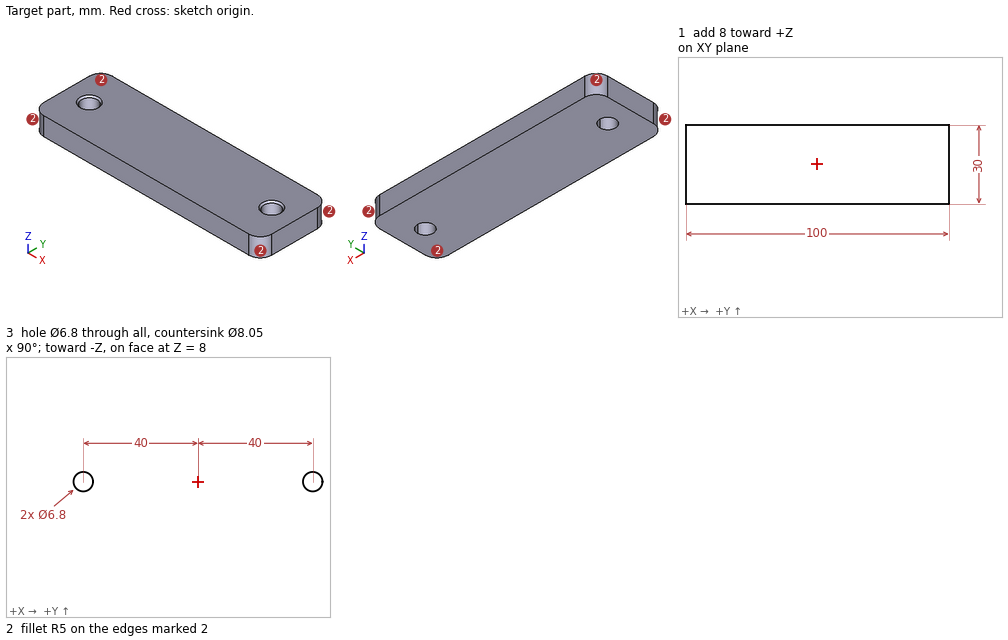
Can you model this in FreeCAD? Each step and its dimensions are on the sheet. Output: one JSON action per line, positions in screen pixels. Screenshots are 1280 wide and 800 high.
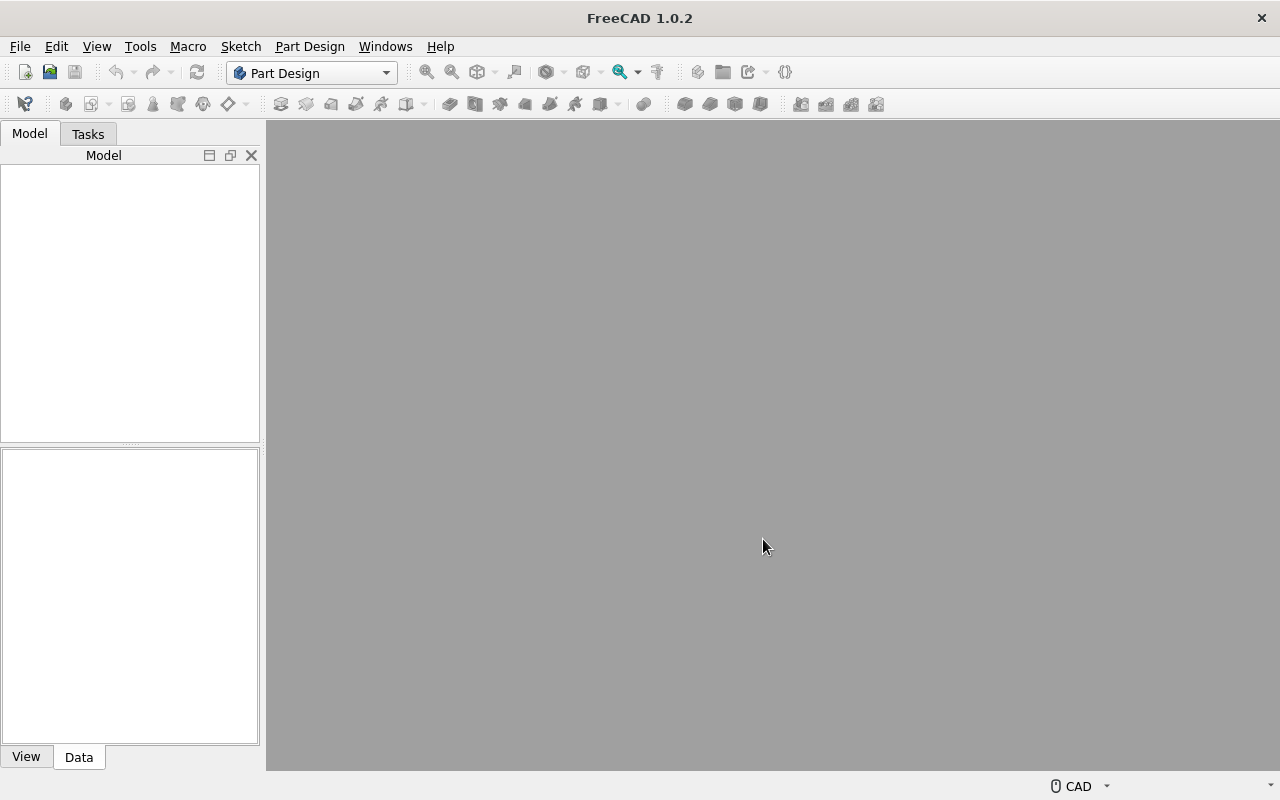
{"action": "left_click", "coordinate": [25, 72]}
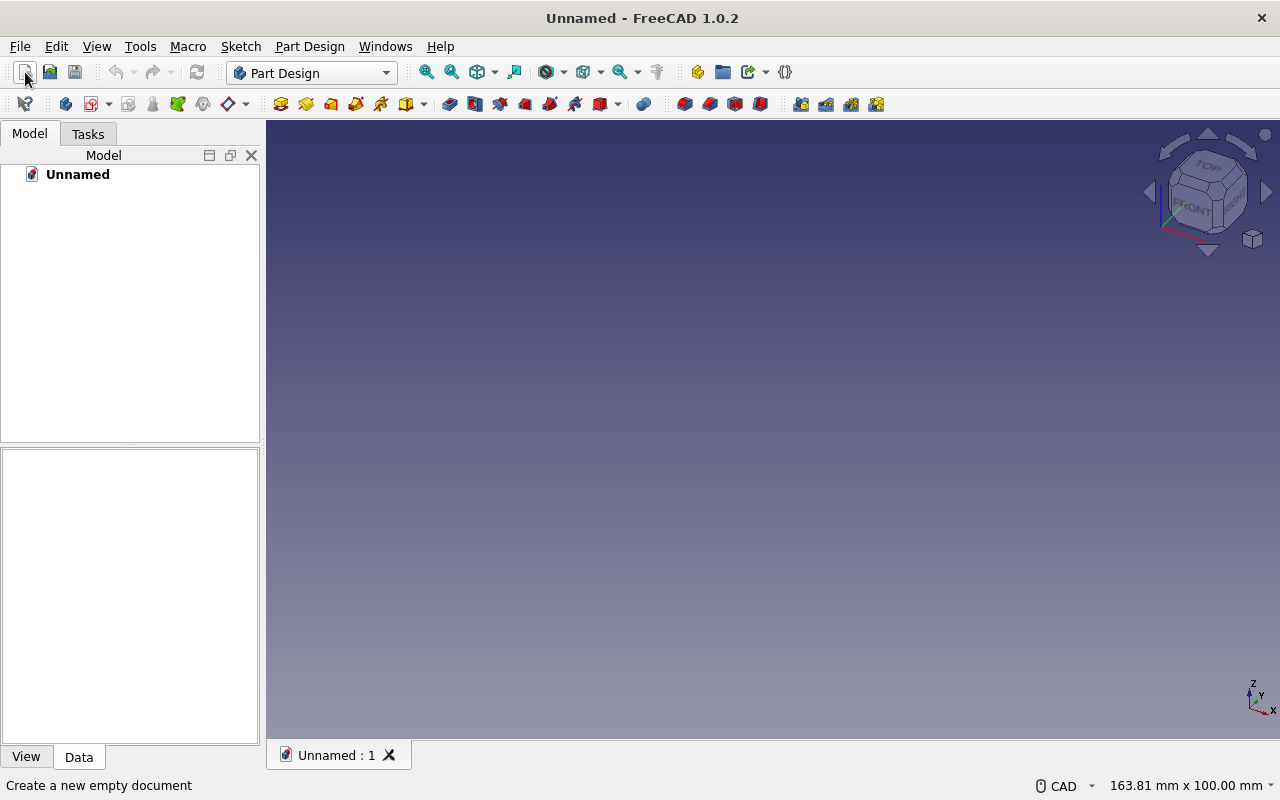
{"action": "left_click", "coordinate": [90, 104]}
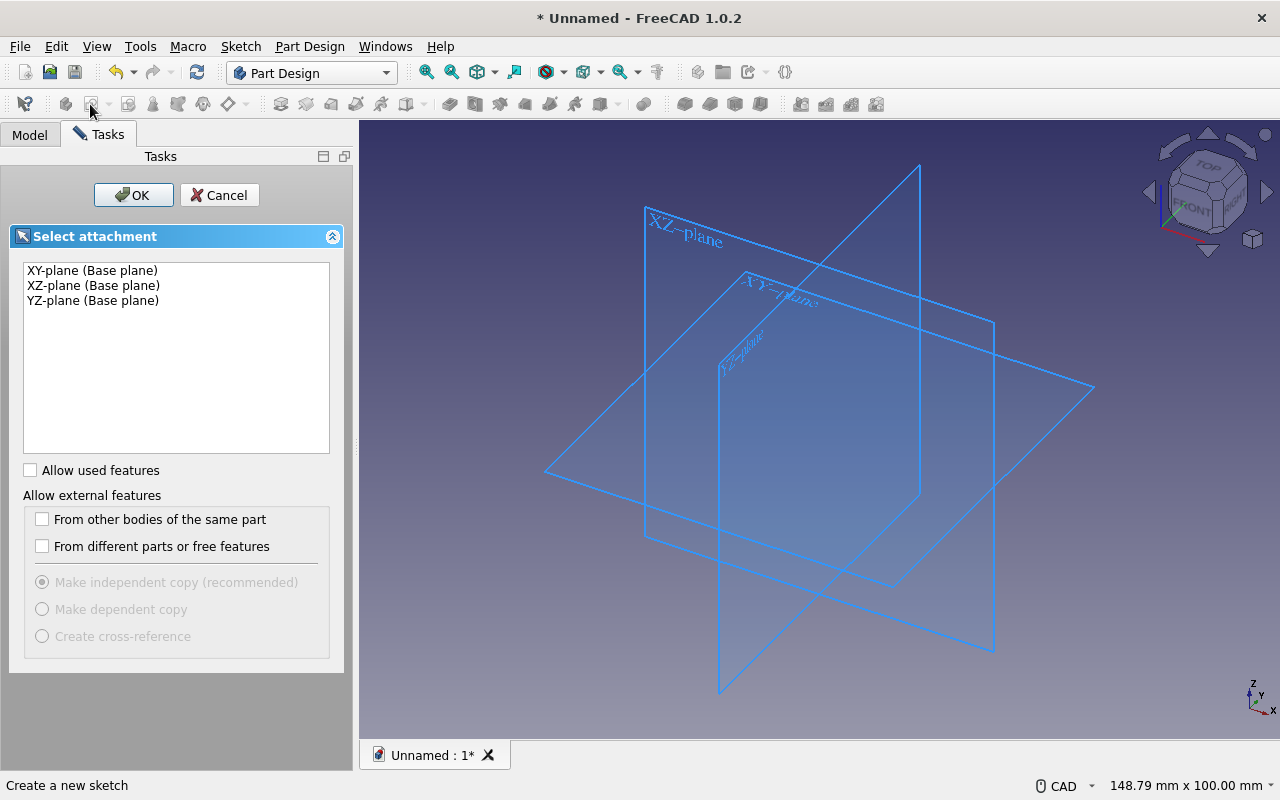
{"action": "left_click", "coordinate": [84, 270]}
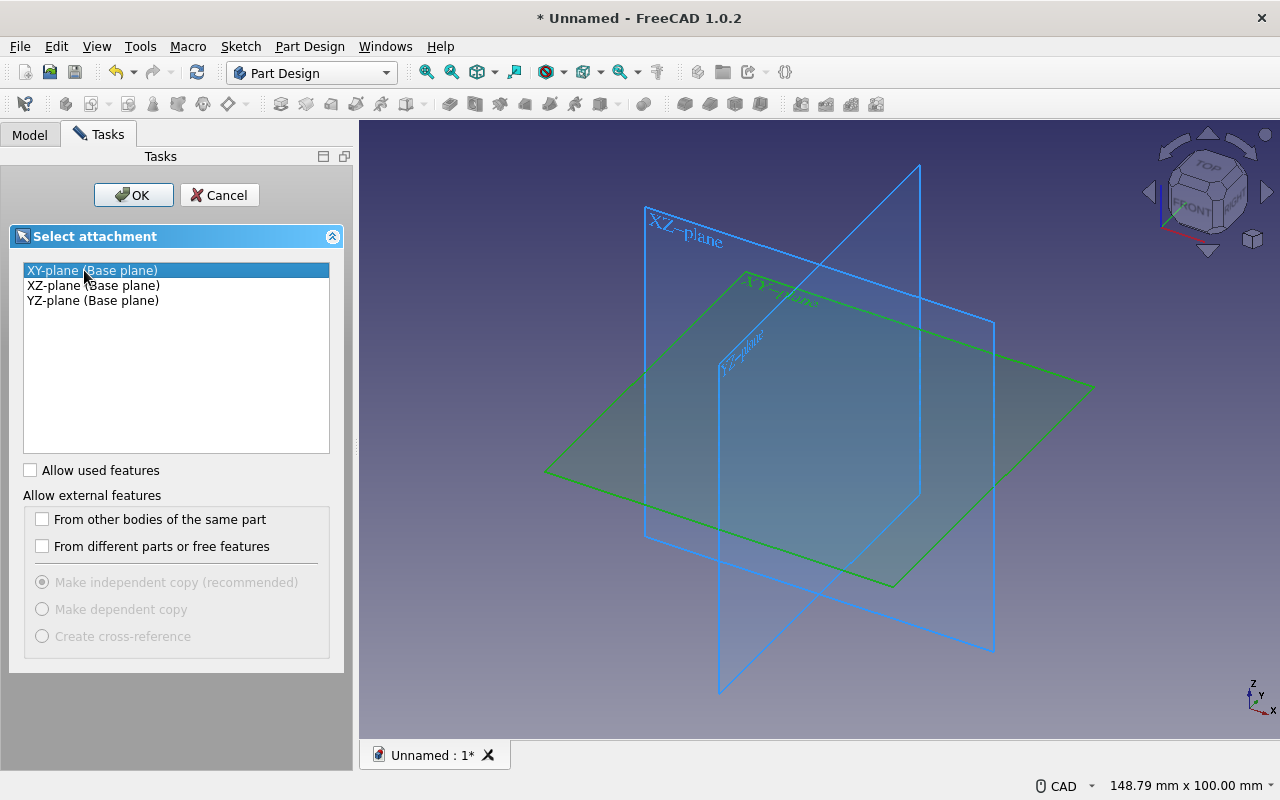
{"action": "left_click", "coordinate": [134, 195]}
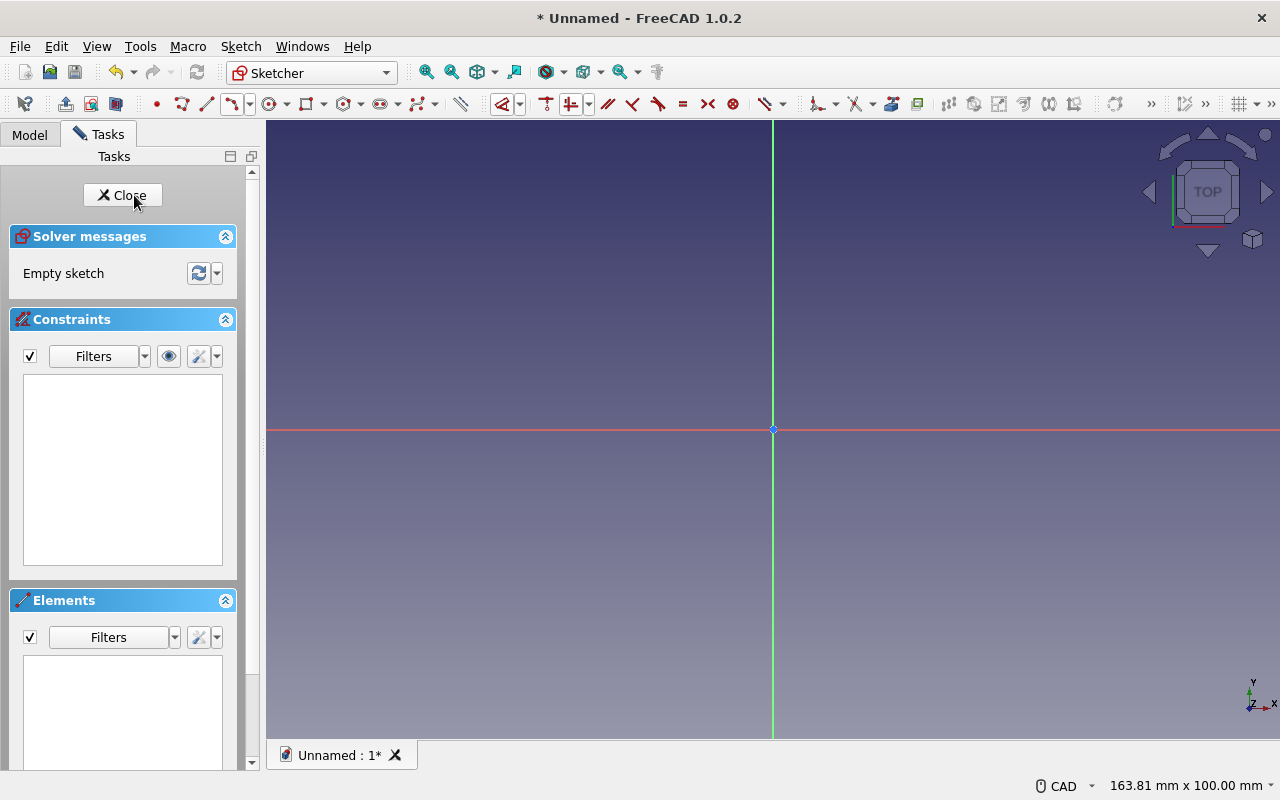
{"action": "key", "text": "g v"}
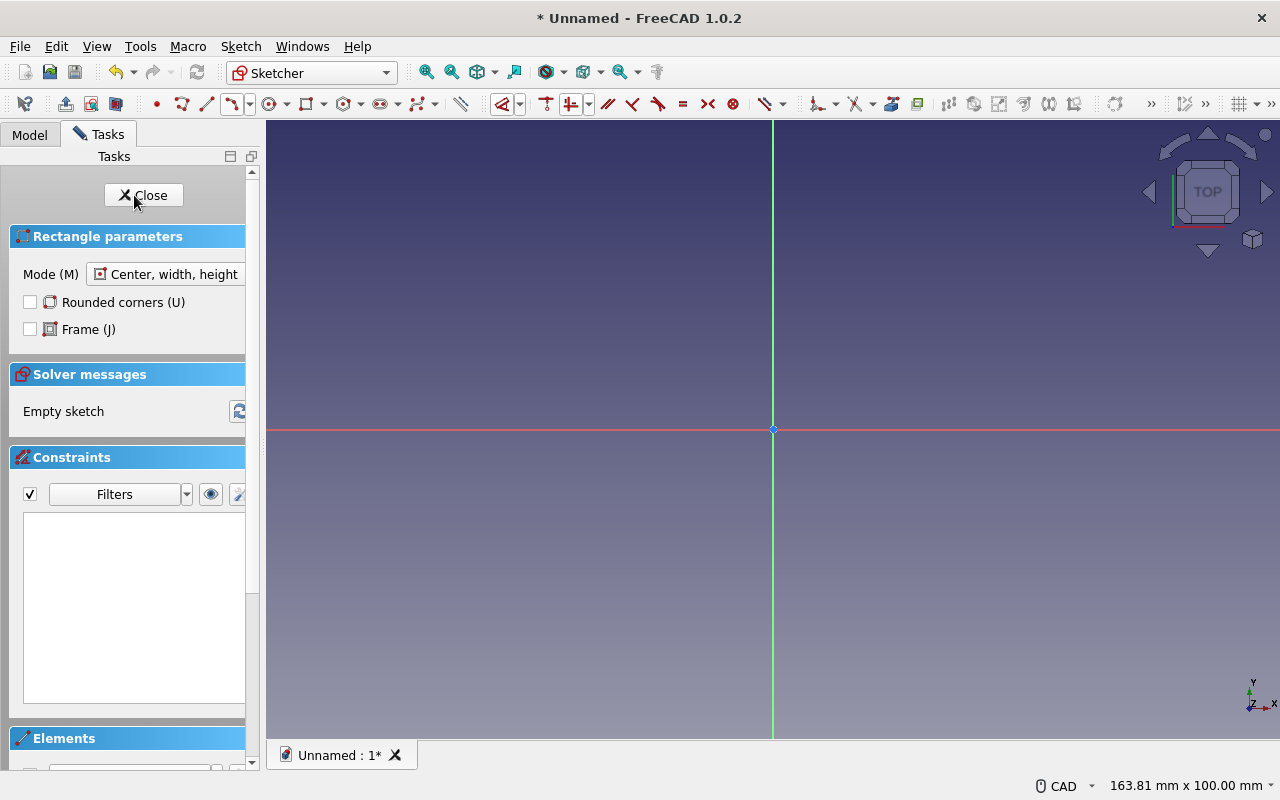
{"action": "left_click", "coordinate": [773, 430]}
{"action": "left_click", "coordinate": [1082, 337]}
{"action": "key", "text": "Escape"}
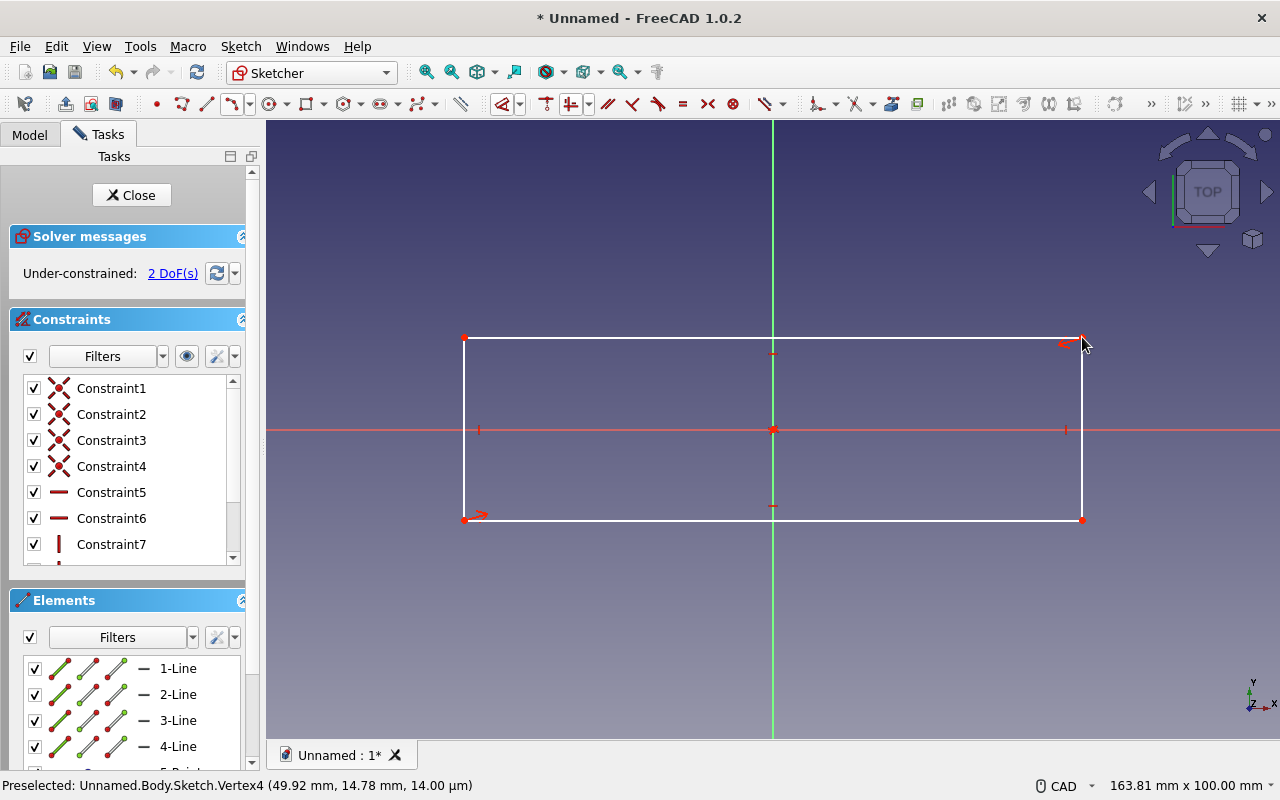
{"action": "left_click", "coordinate": [1082, 466]}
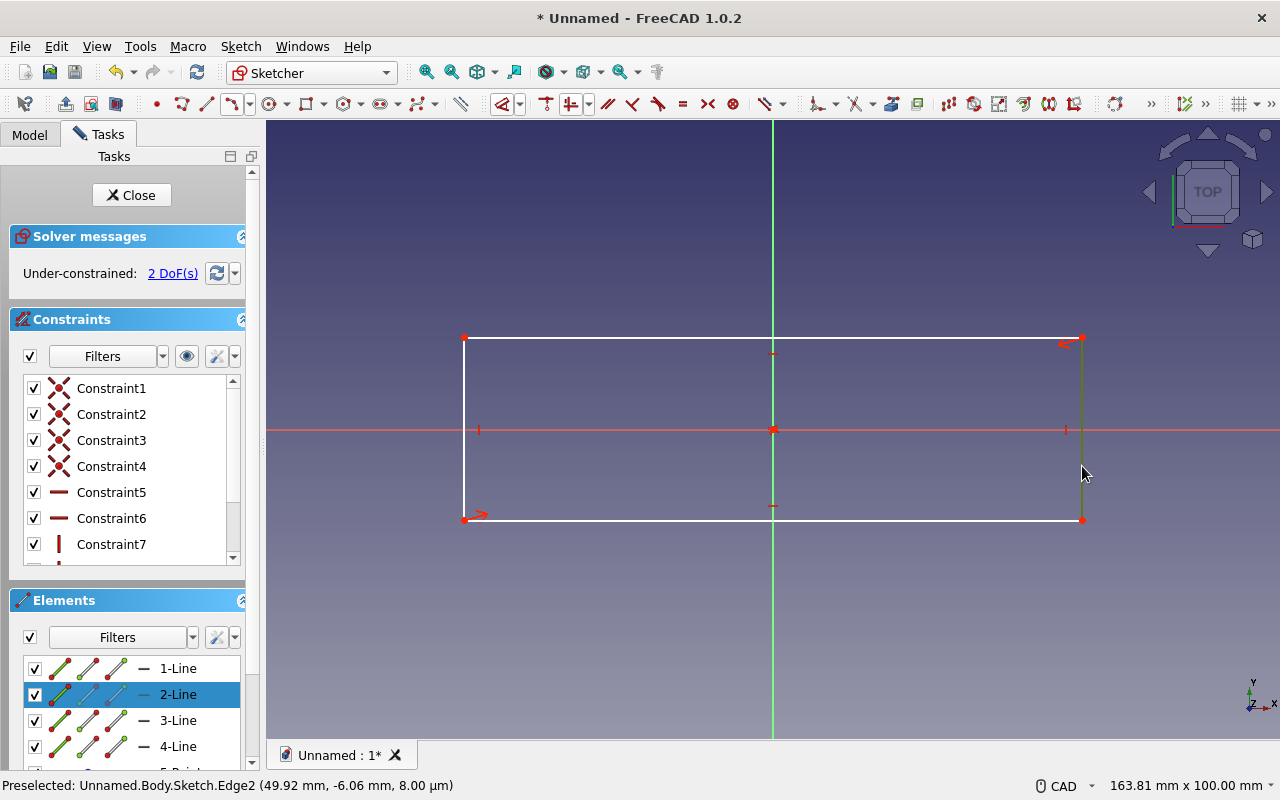
{"action": "left_click", "coordinate": [520, 104]}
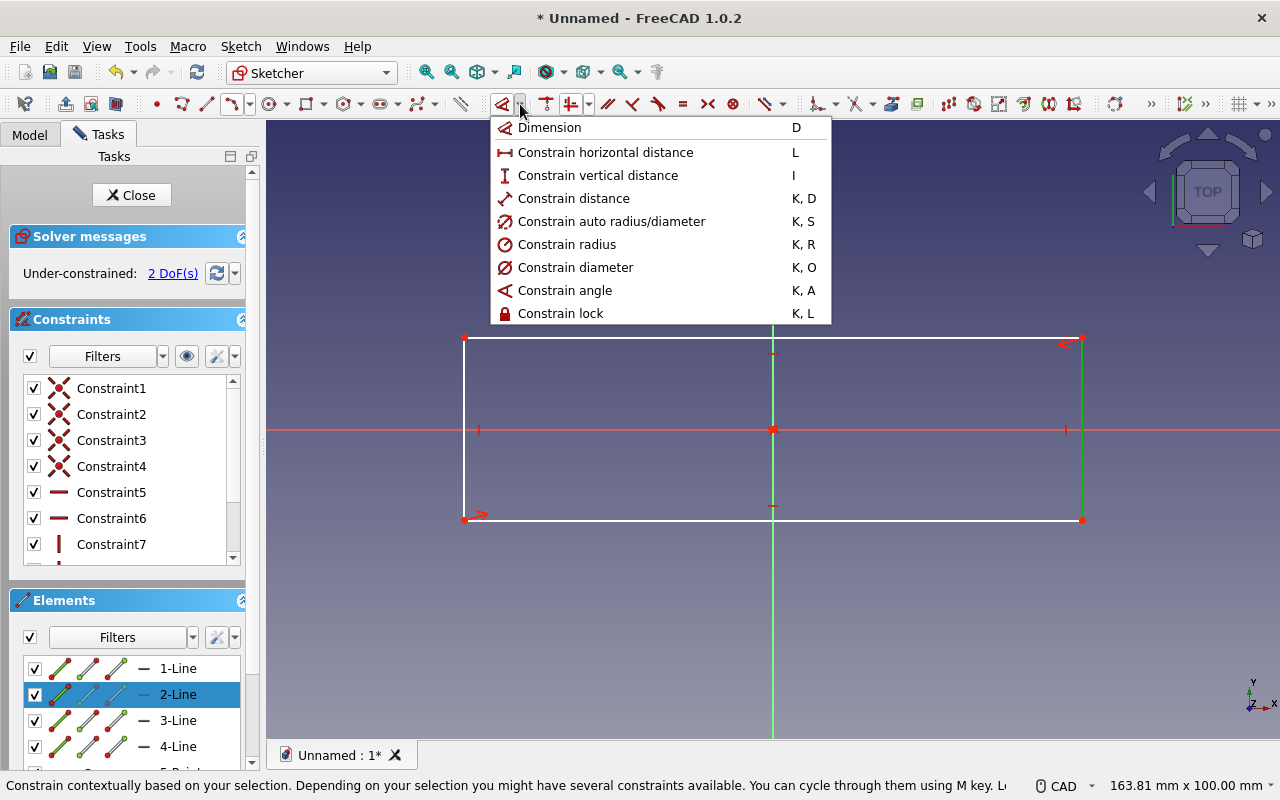
{"action": "left_click", "coordinate": [661, 176]}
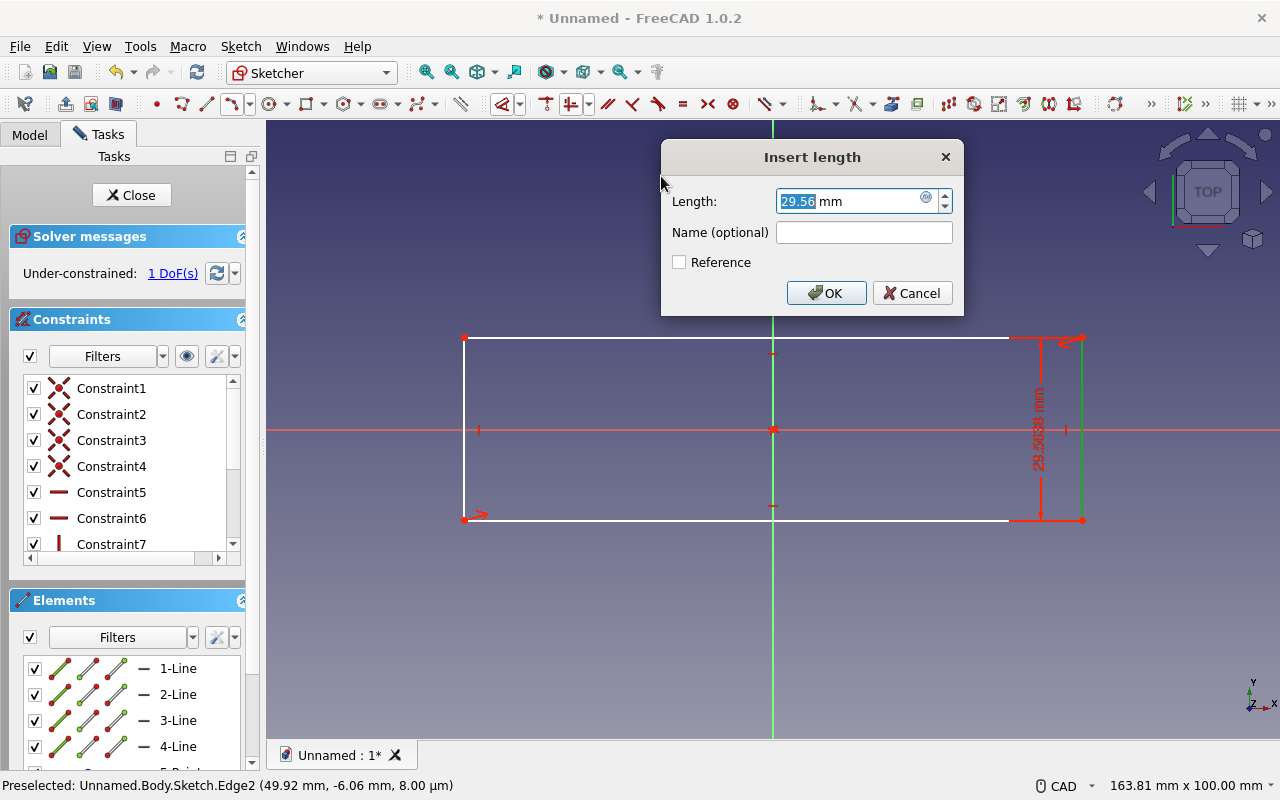
{"action": "type", "text": "30"}
{"action": "key", "text": "Return"}